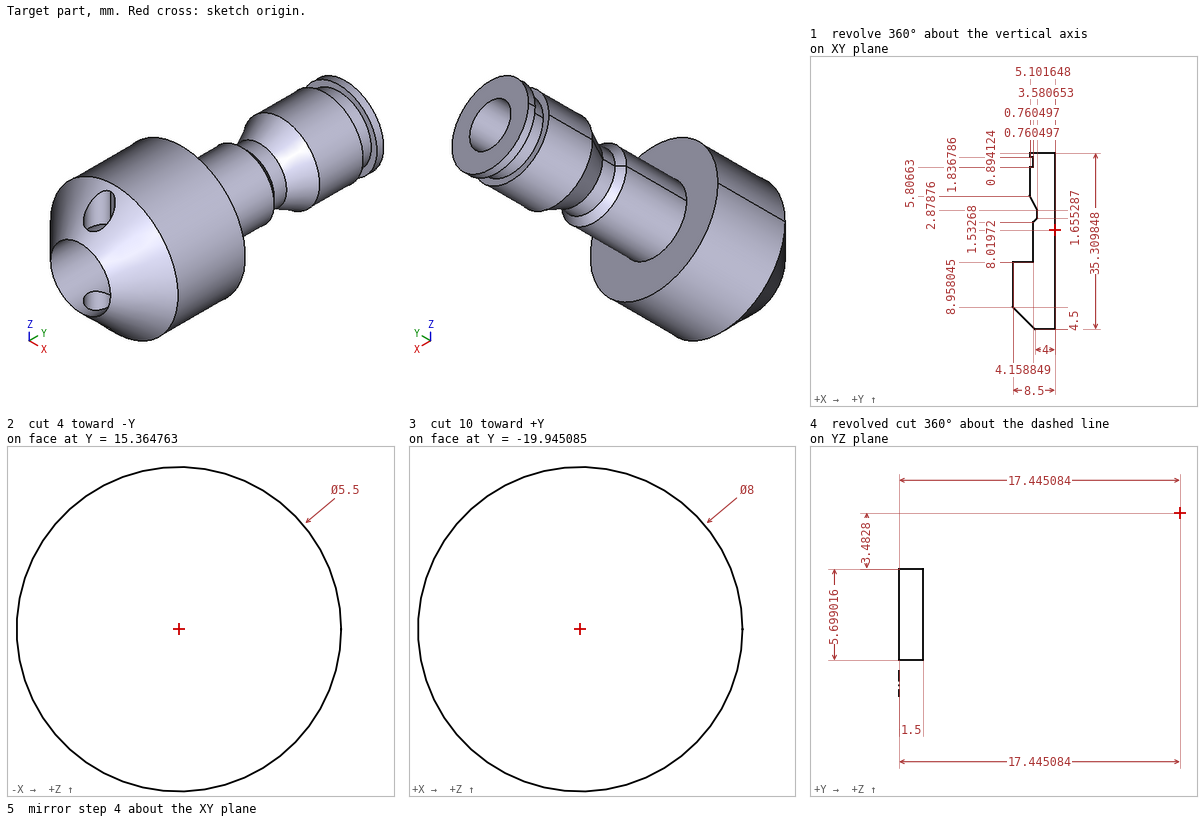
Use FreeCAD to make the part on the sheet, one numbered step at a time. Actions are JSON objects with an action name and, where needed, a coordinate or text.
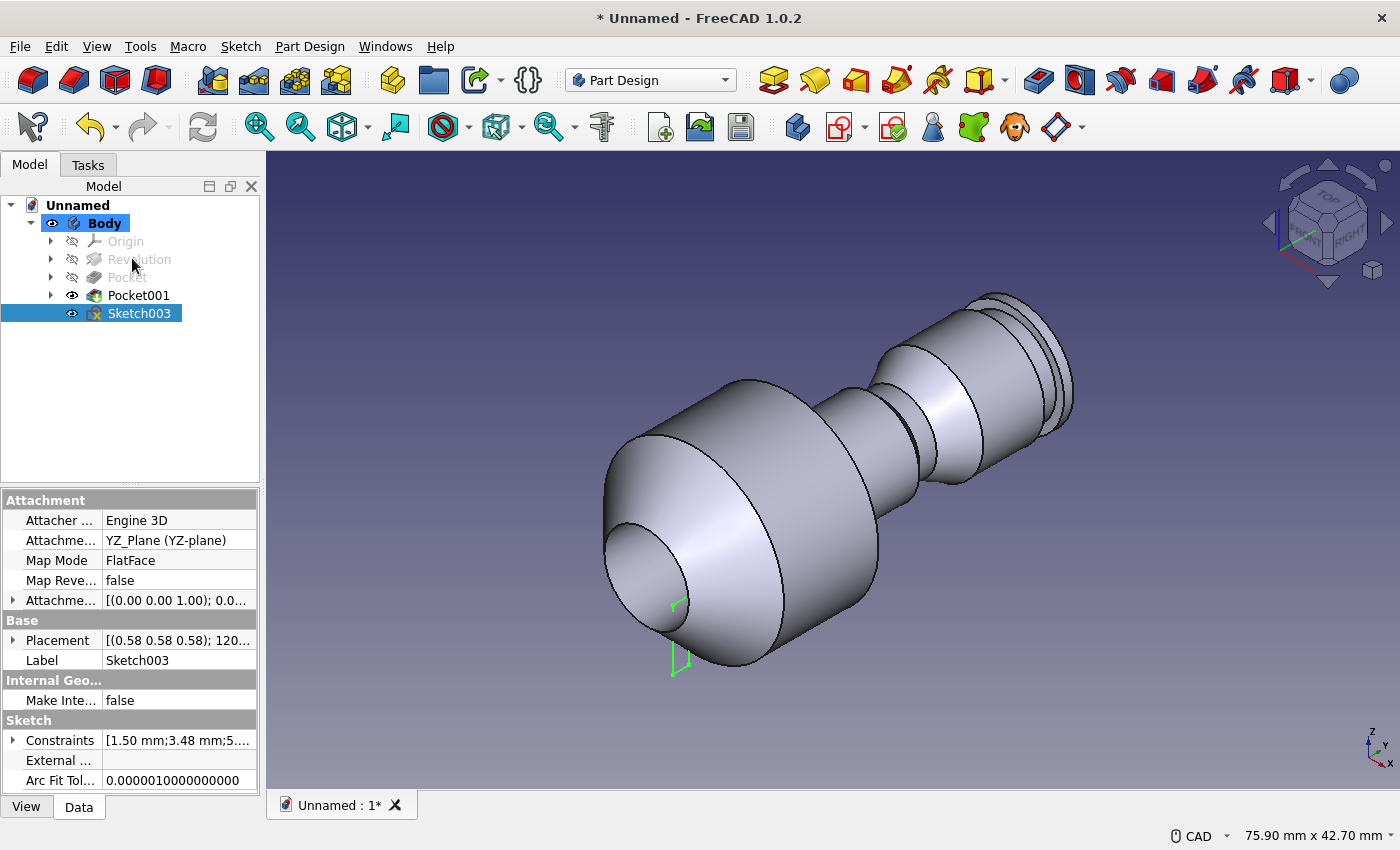
{"action": "left_click", "coordinate": [1121, 80]}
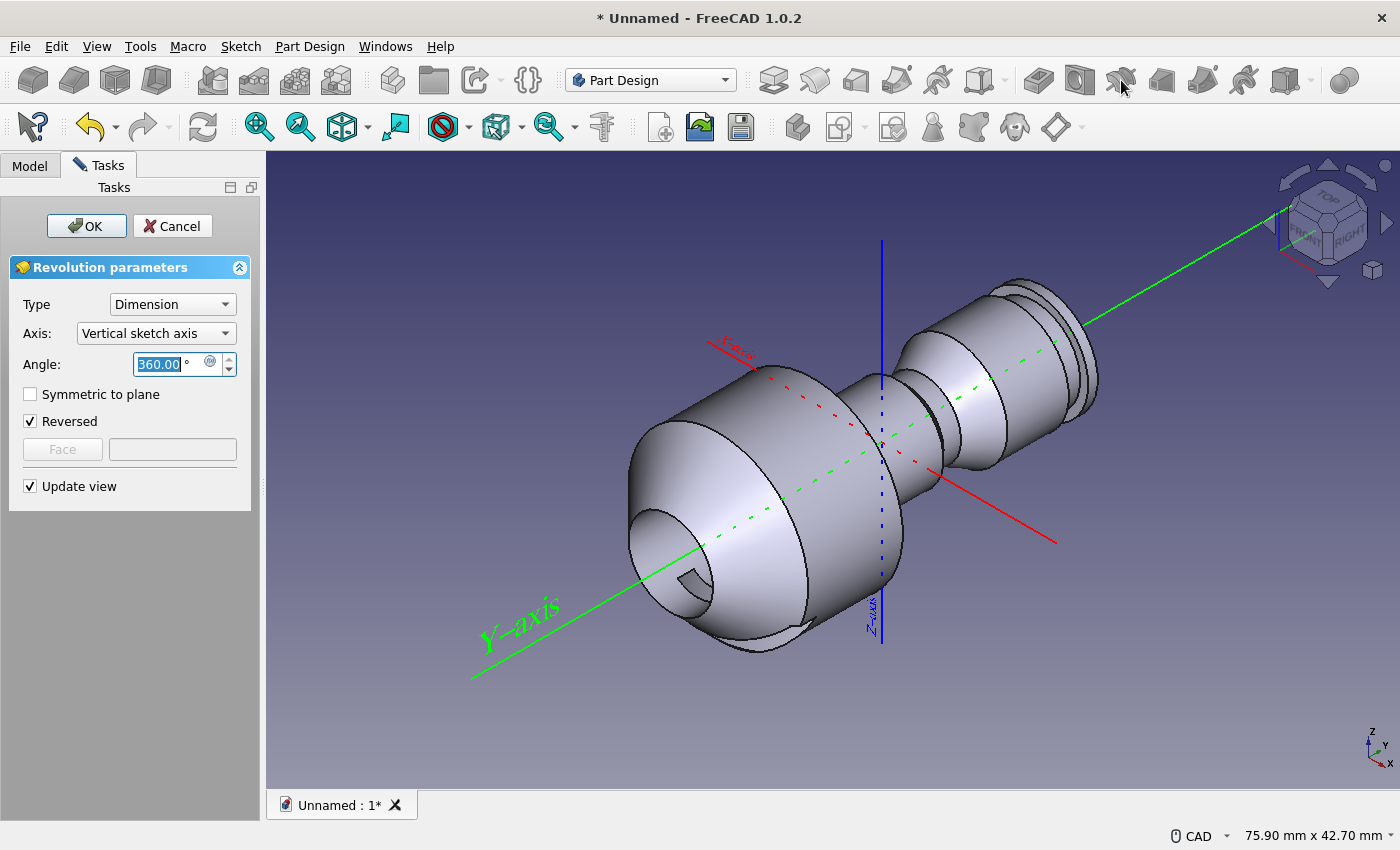
{"action": "left_click", "coordinate": [157, 334]}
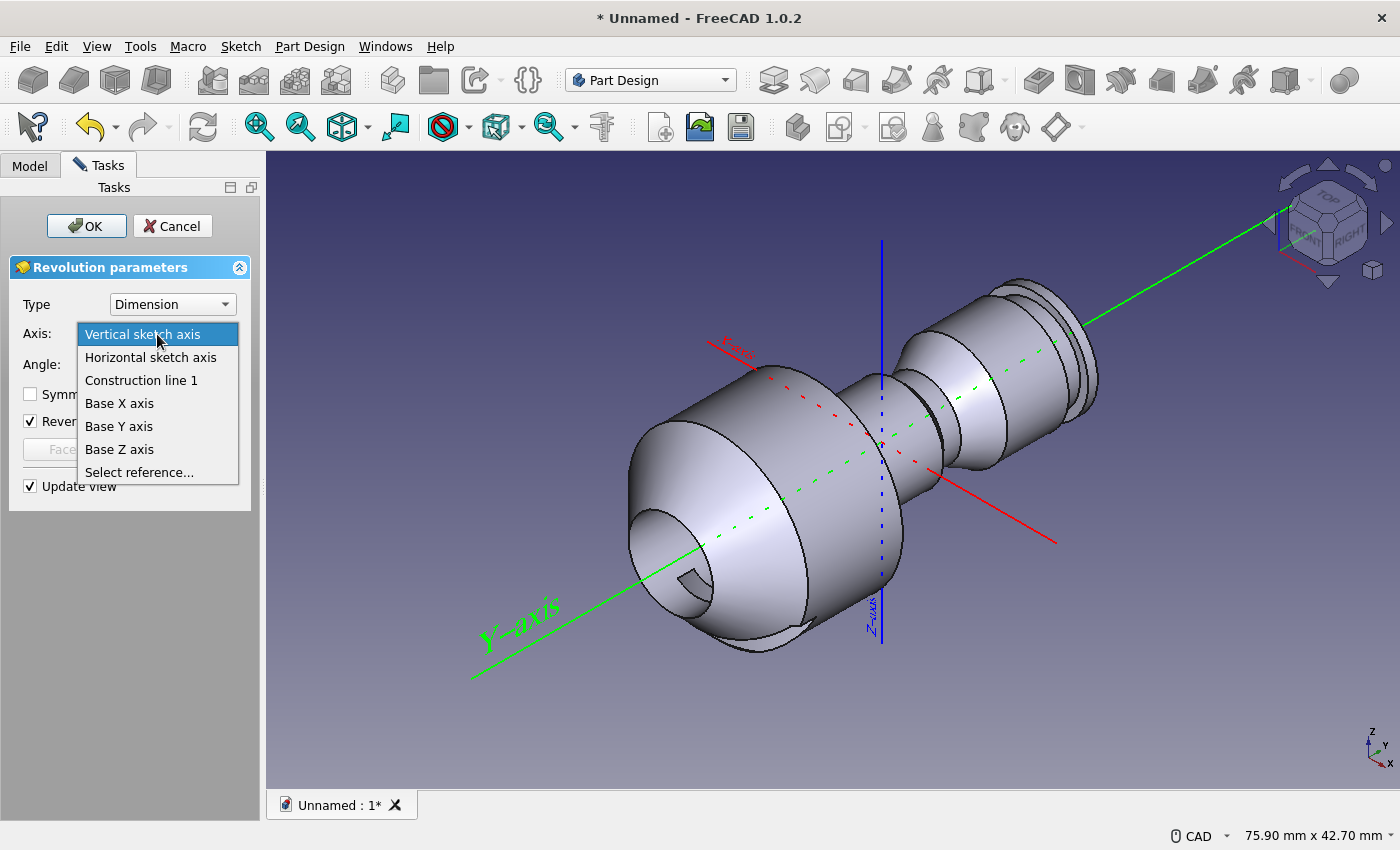
{"action": "left_click", "coordinate": [156, 380]}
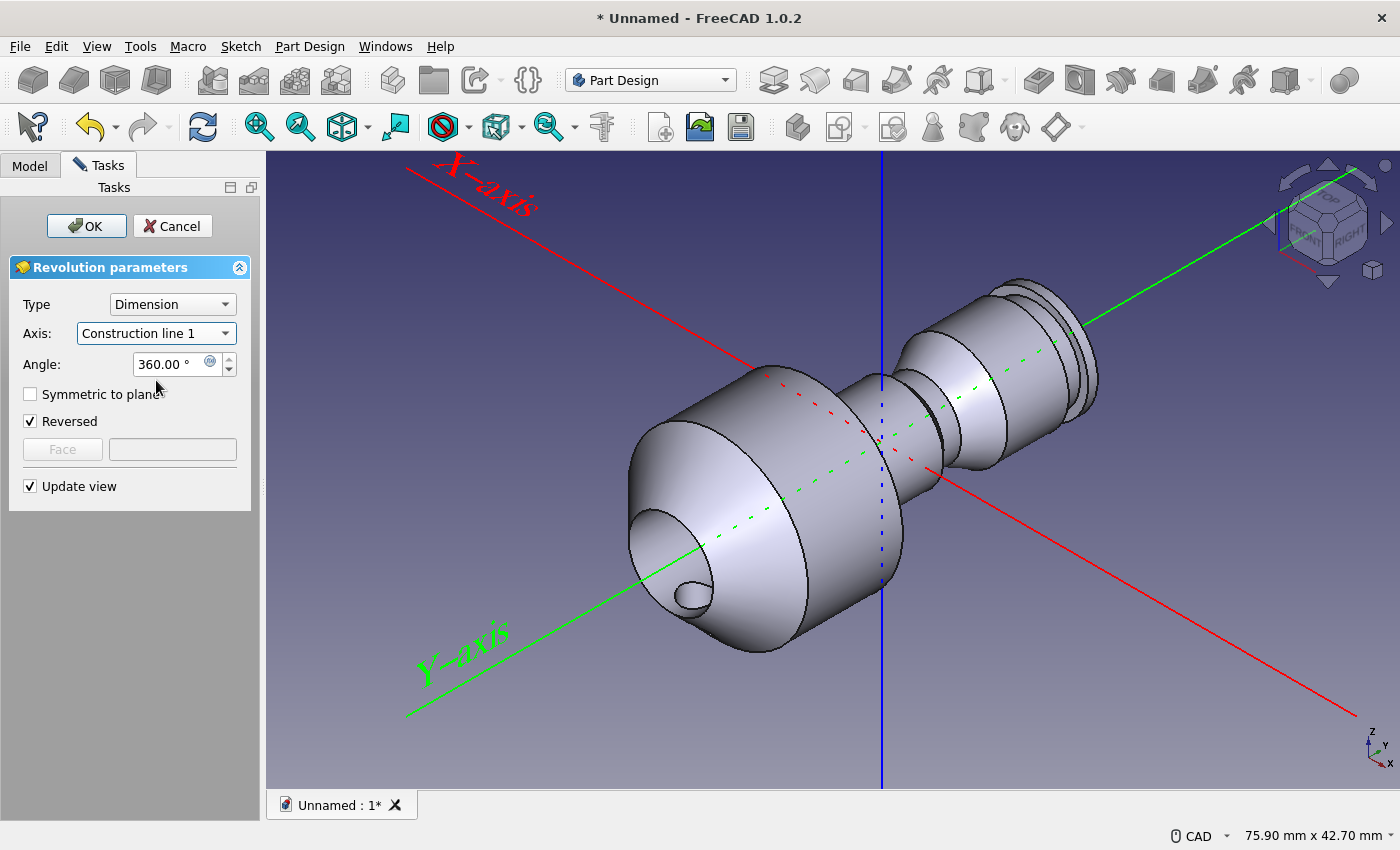
{"action": "left_click", "coordinate": [87, 226]}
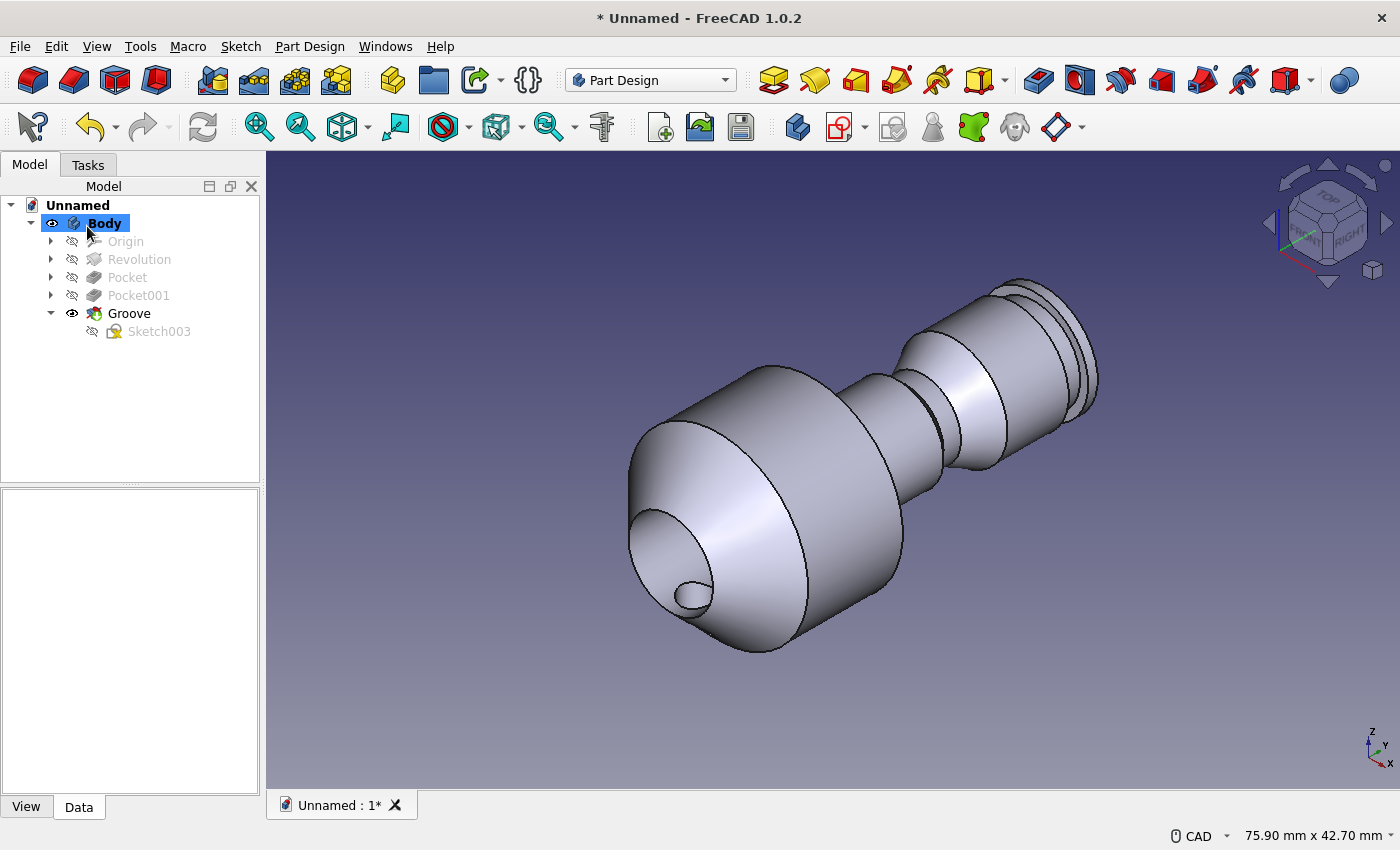
{"action": "left_click", "coordinate": [117, 313]}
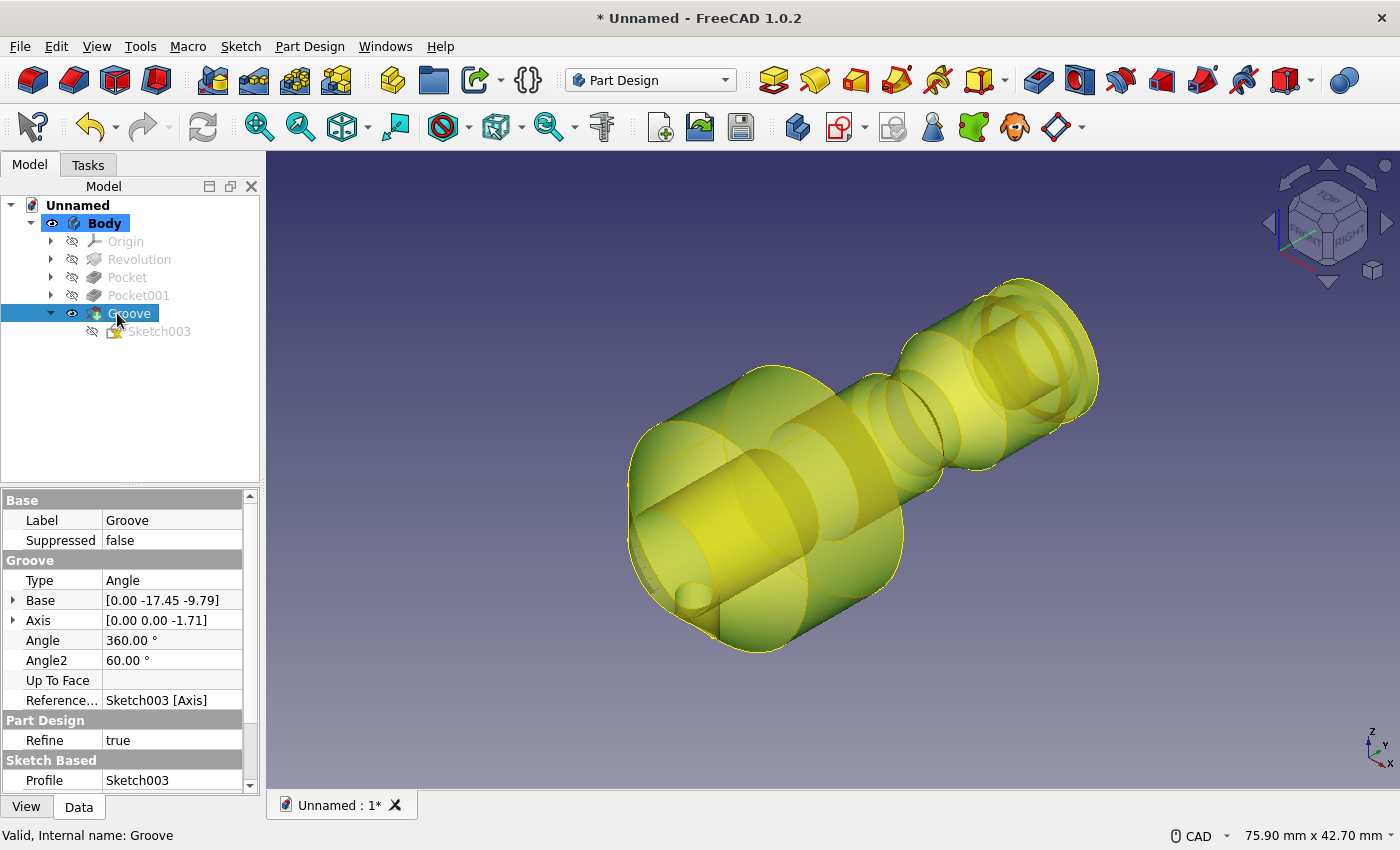
{"action": "left_click", "coordinate": [213, 80]}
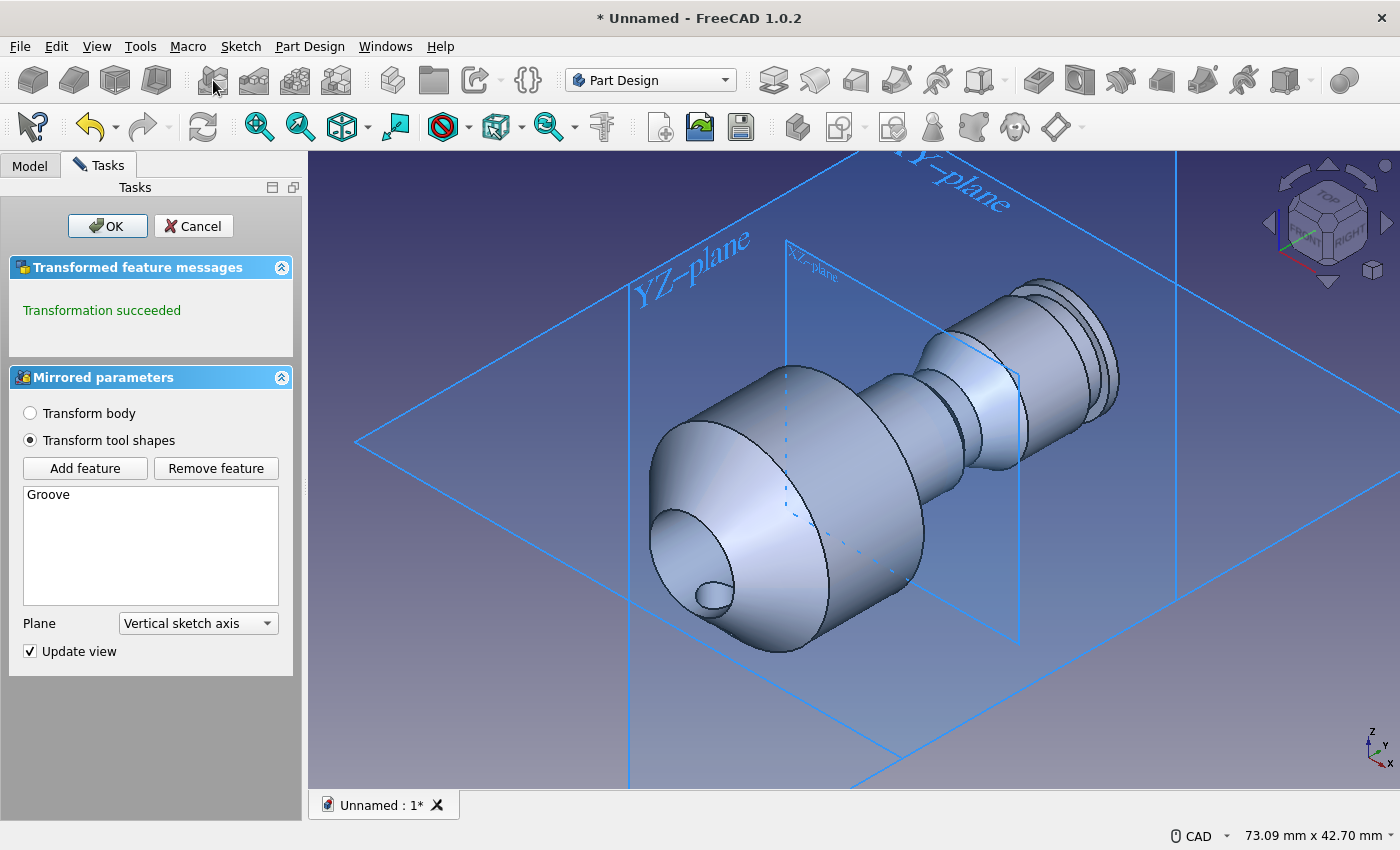
{"action": "left_click", "coordinate": [199, 624]}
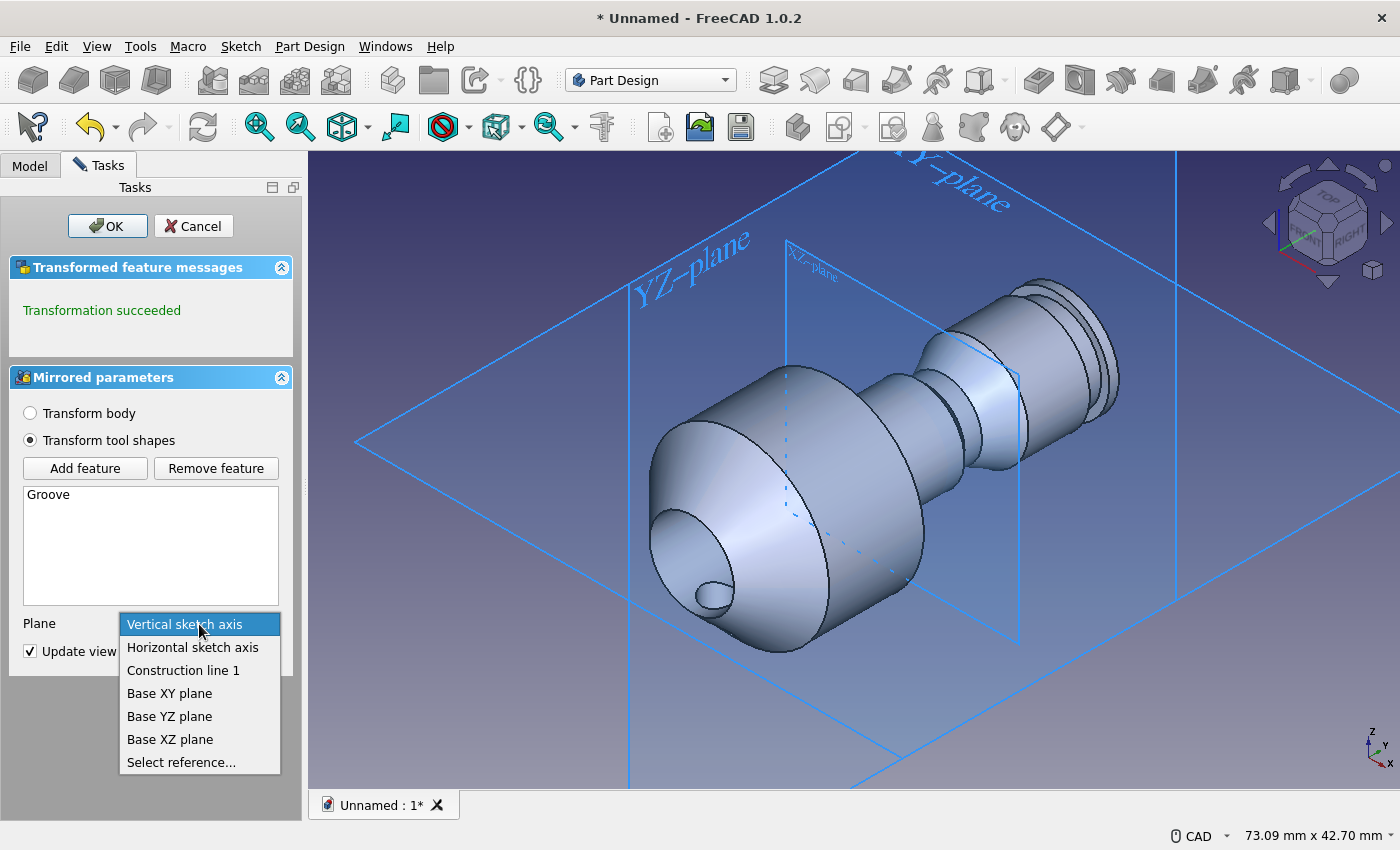
{"action": "left_click", "coordinate": [198, 694]}